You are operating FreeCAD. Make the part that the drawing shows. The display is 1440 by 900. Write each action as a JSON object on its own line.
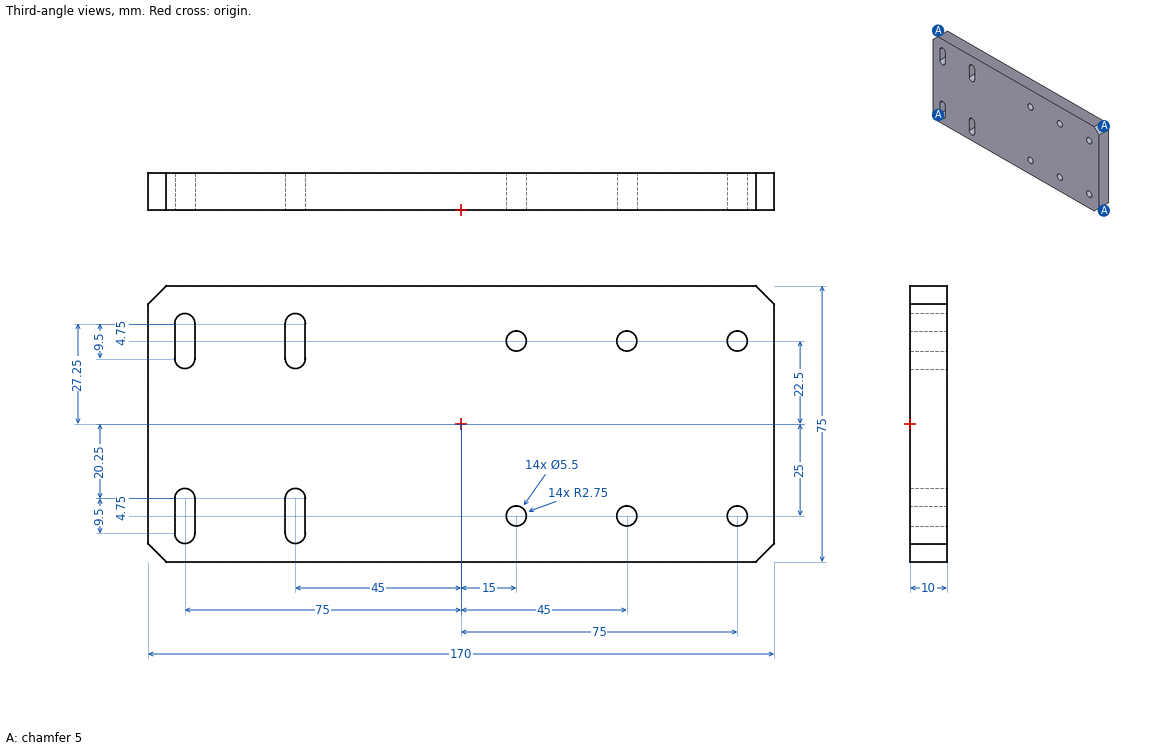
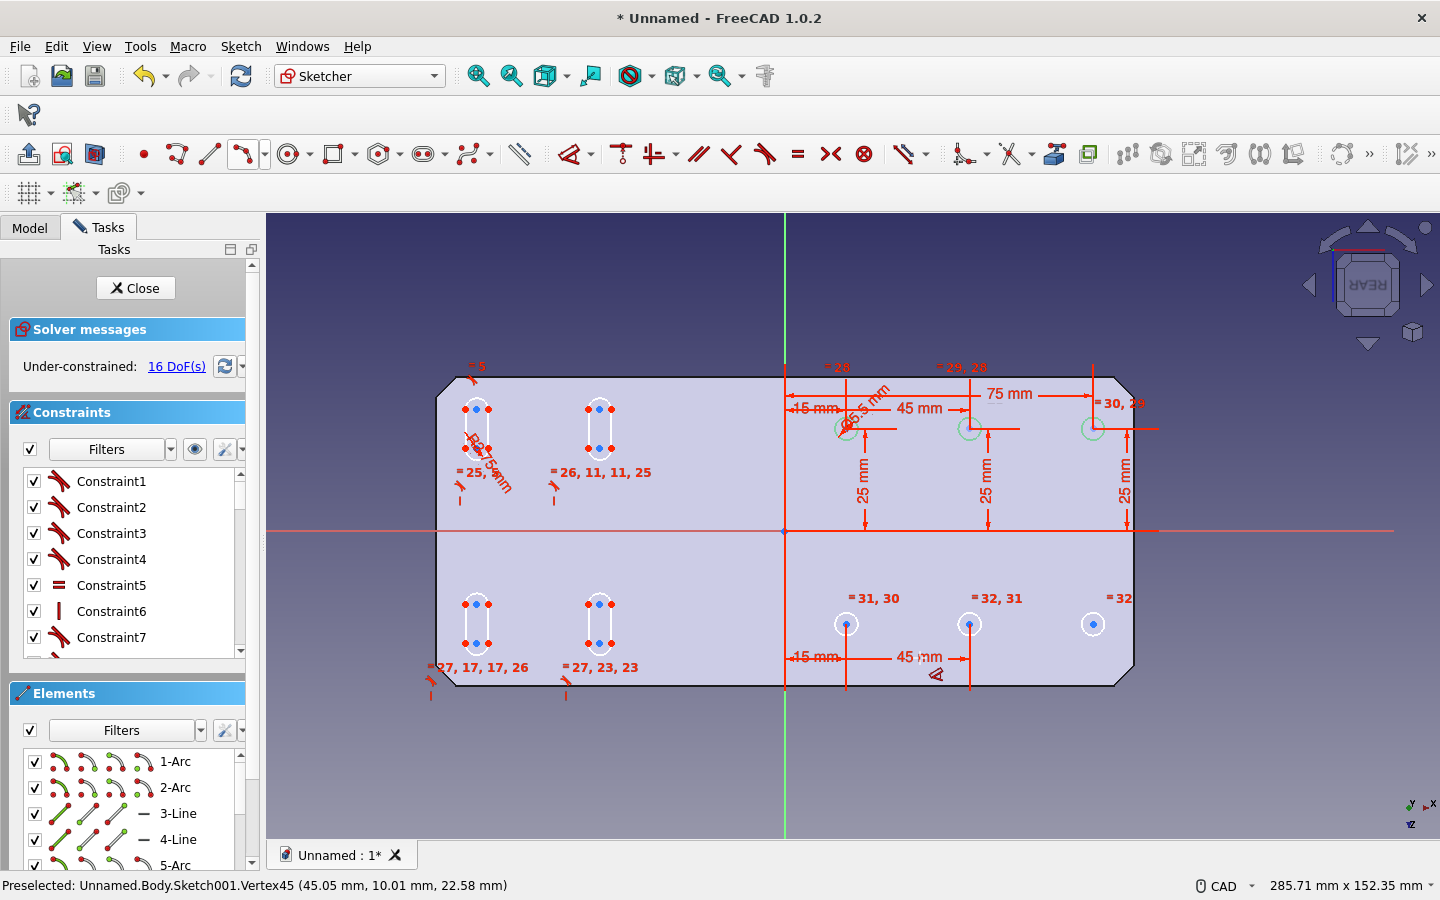
{"action": "left_click", "coordinate": [1093, 624]}
{"action": "left_click", "coordinate": [1010, 658]}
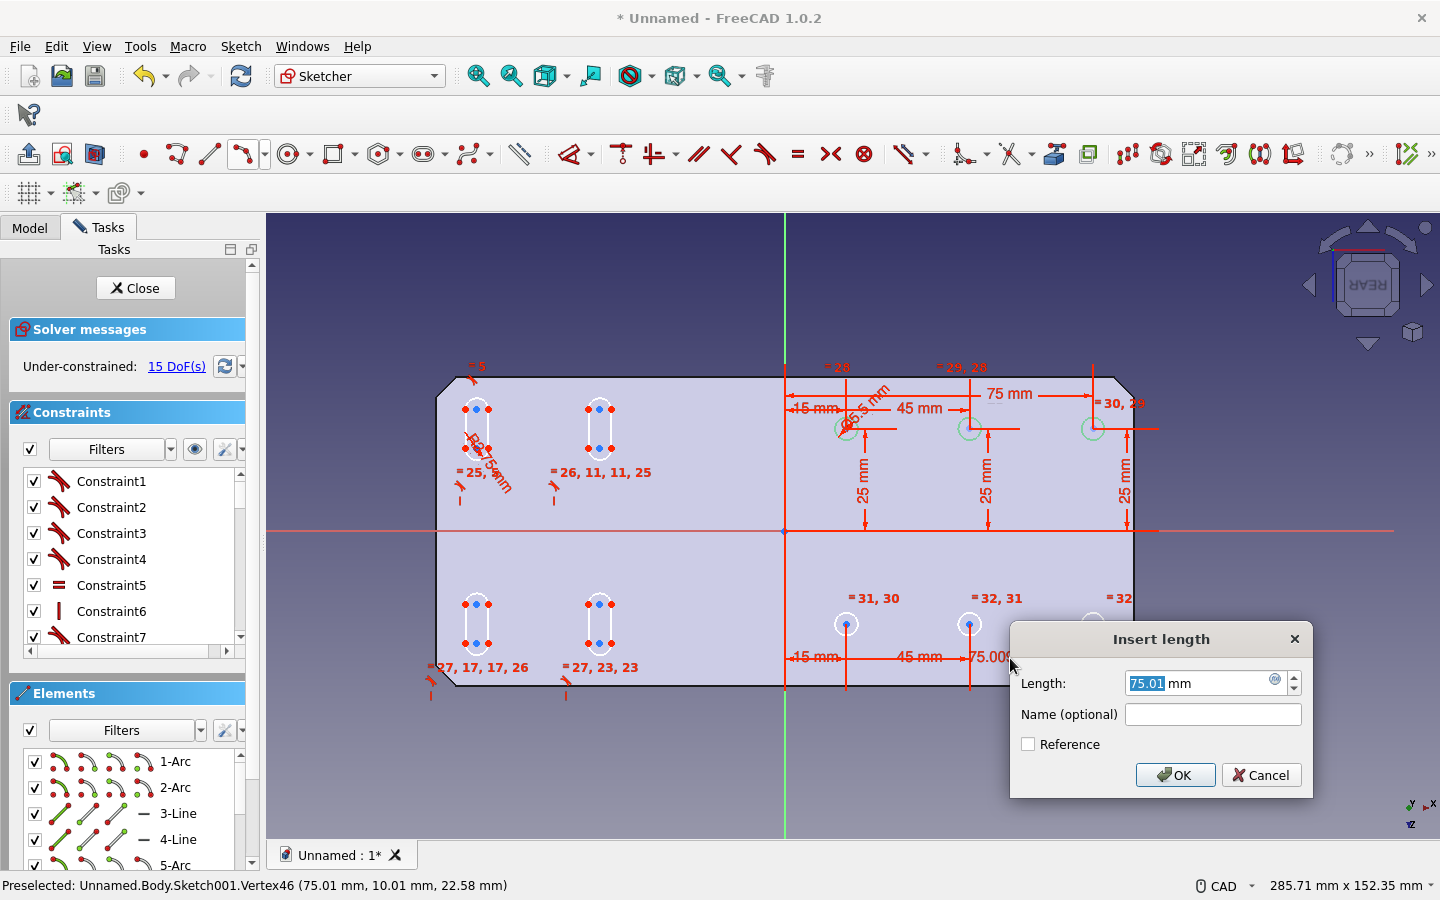
{"action": "type", "text": "75"}
{"action": "key", "text": "Return"}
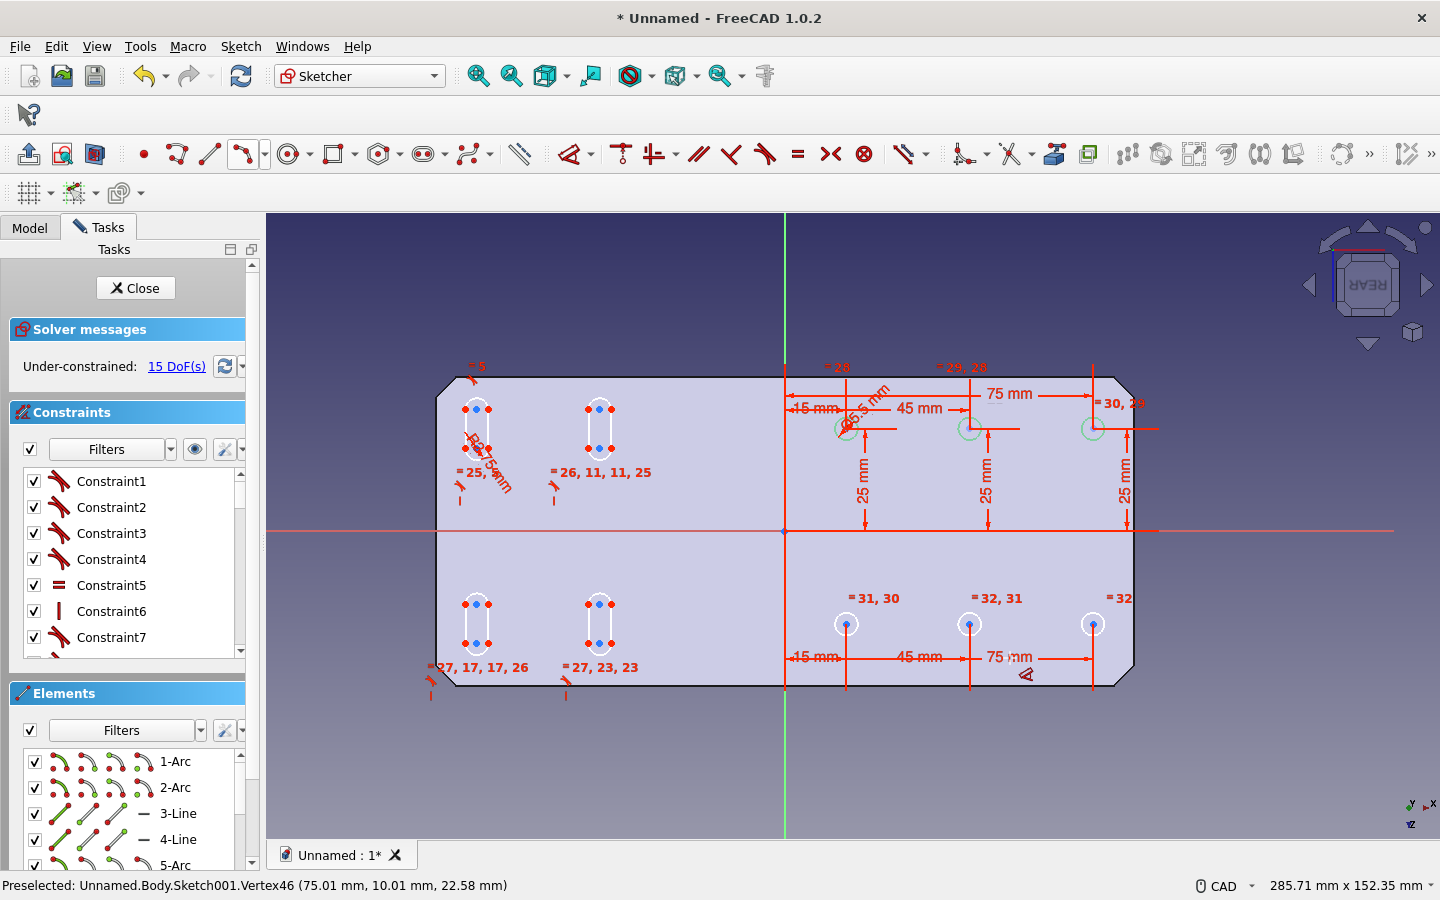
{"action": "left_click", "coordinate": [466, 437]}
{"action": "left_click", "coordinate": [432, 429]}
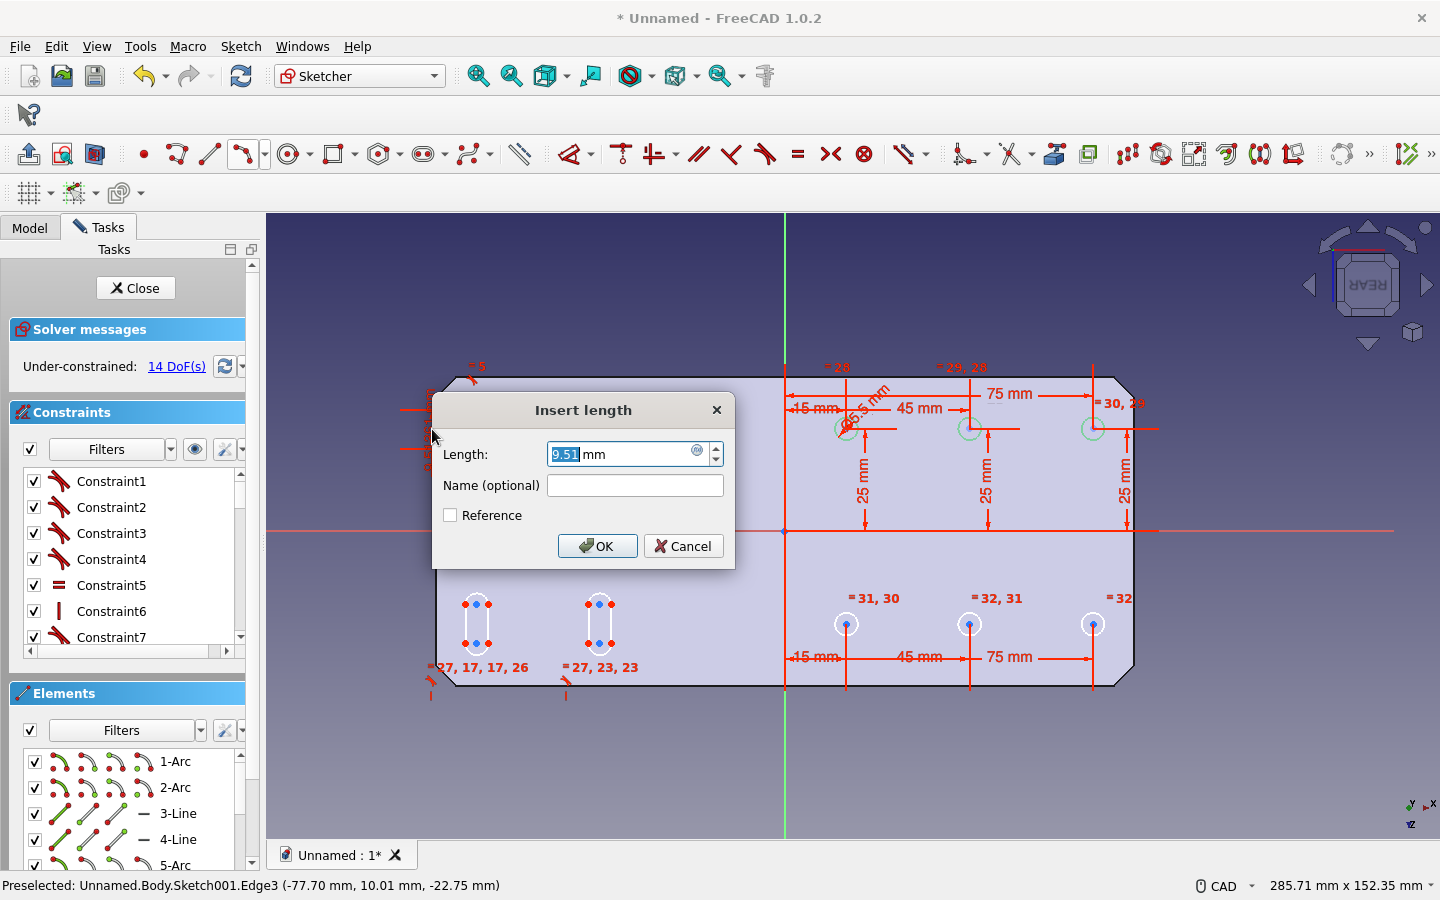
{"action": "type", "text": "9.5"}
{"action": "key", "text": "Return"}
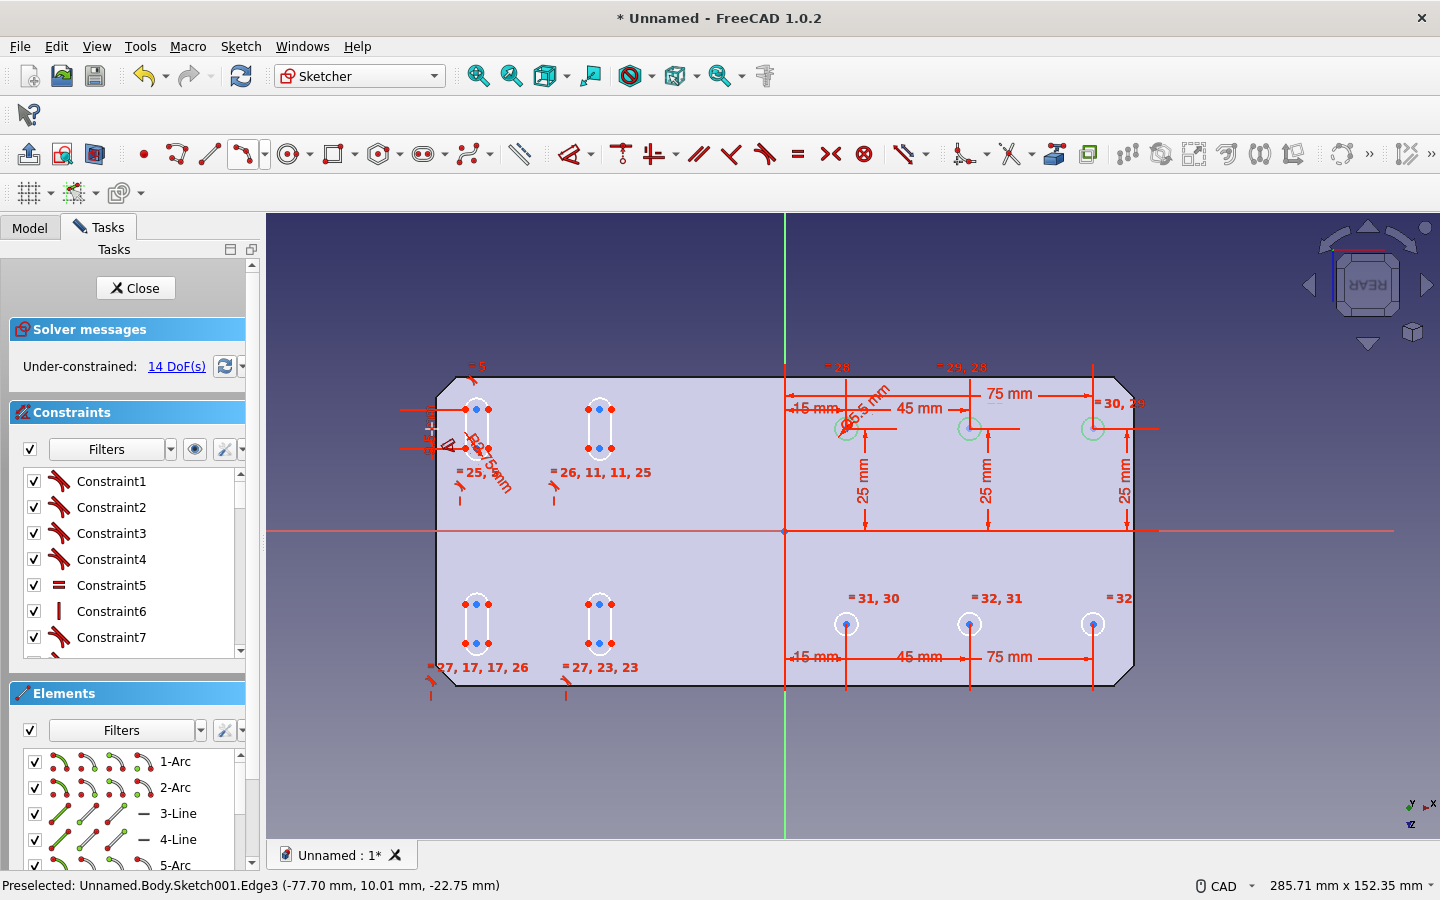
{"action": "left_click", "coordinate": [589, 437]}
{"action": "left_click", "coordinate": [555, 429]}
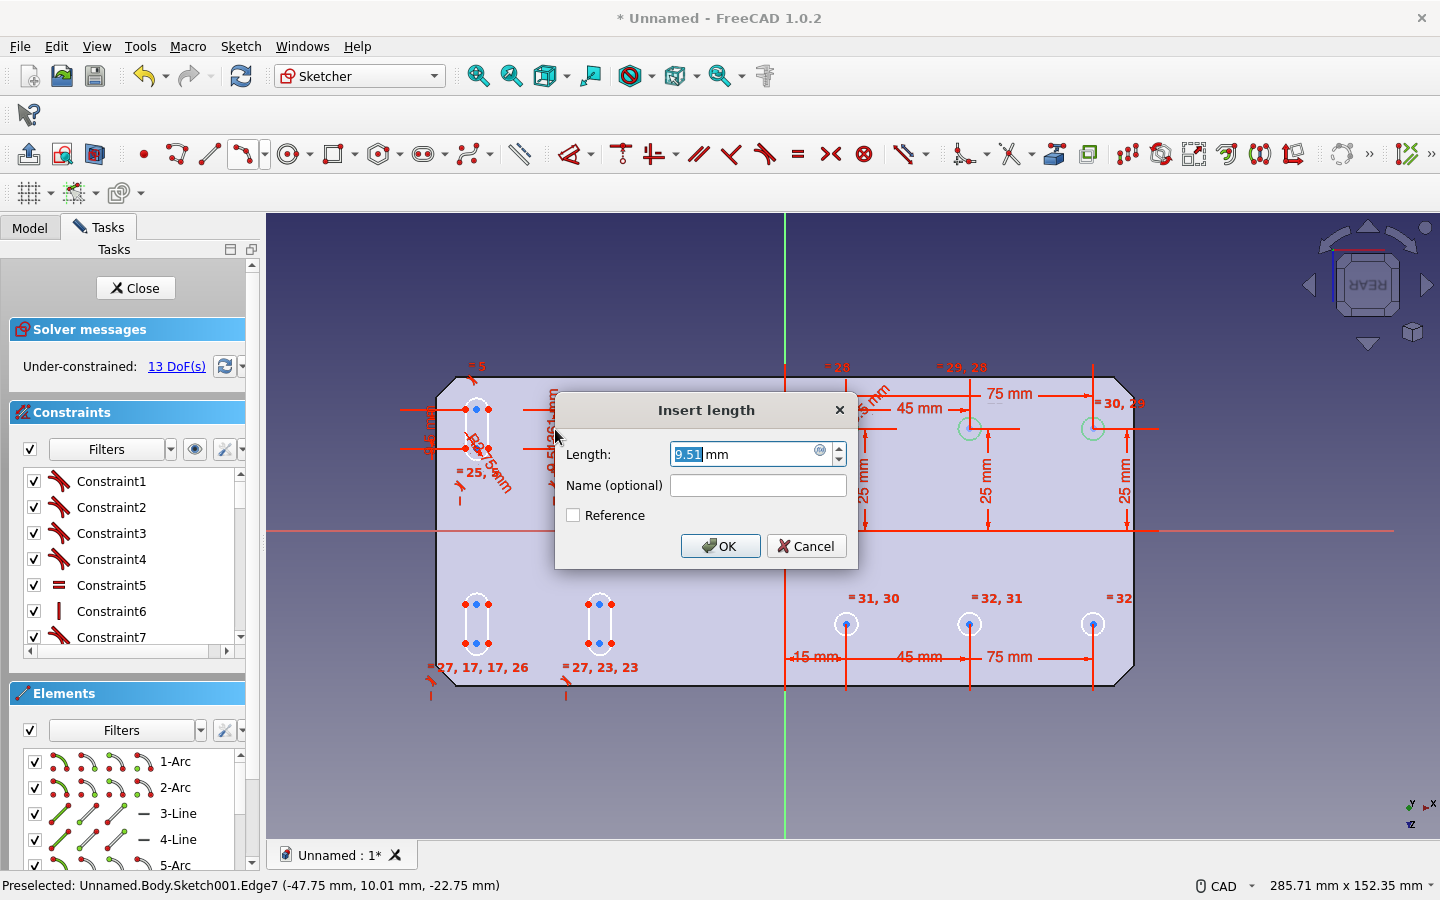
{"action": "type", "text": "9.5"}
{"action": "key", "text": "Return"}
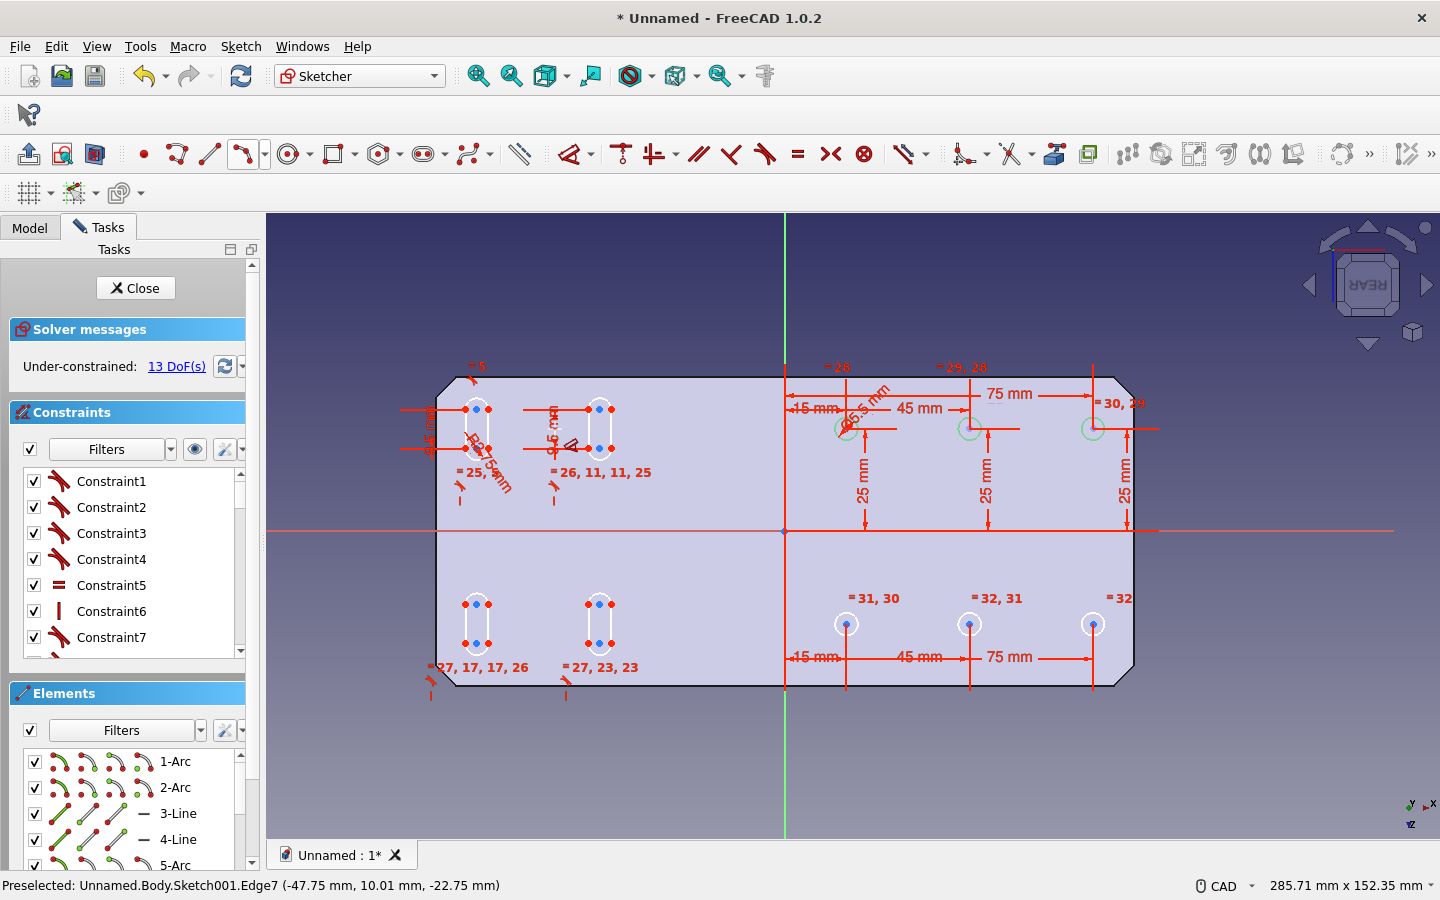
{"action": "left_click", "coordinate": [466, 632]}
{"action": "left_click", "coordinate": [432, 624]}